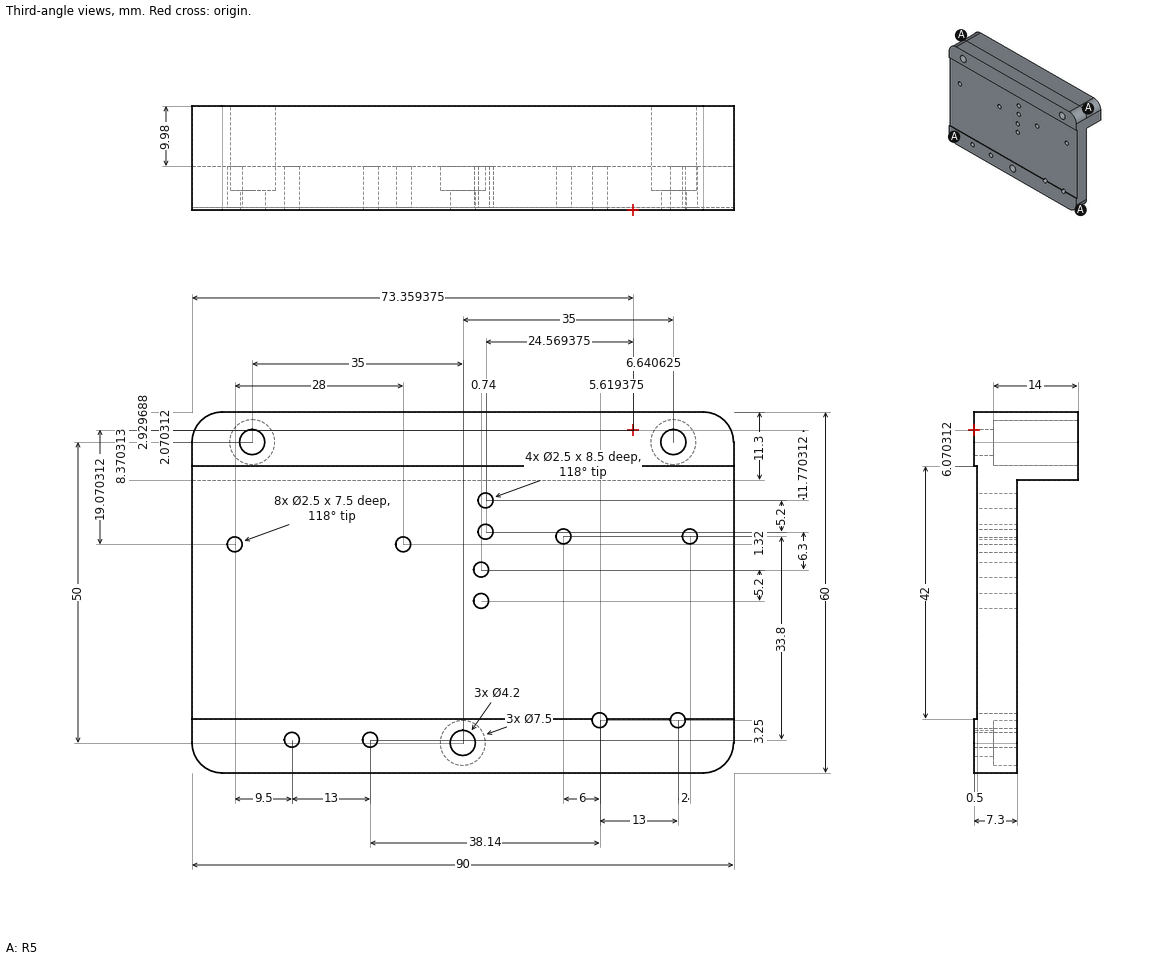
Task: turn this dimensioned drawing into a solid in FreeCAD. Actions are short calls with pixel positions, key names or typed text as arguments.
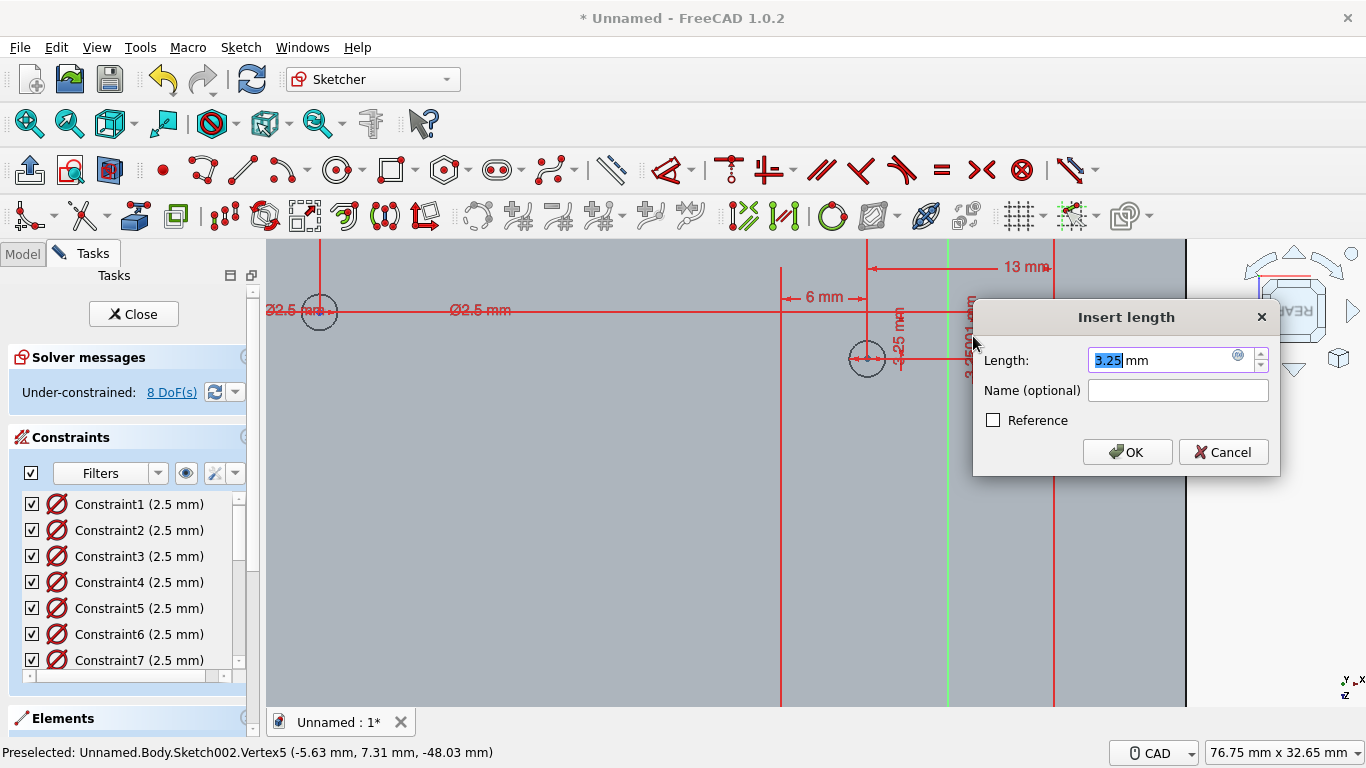
text(3.25)
key(Return)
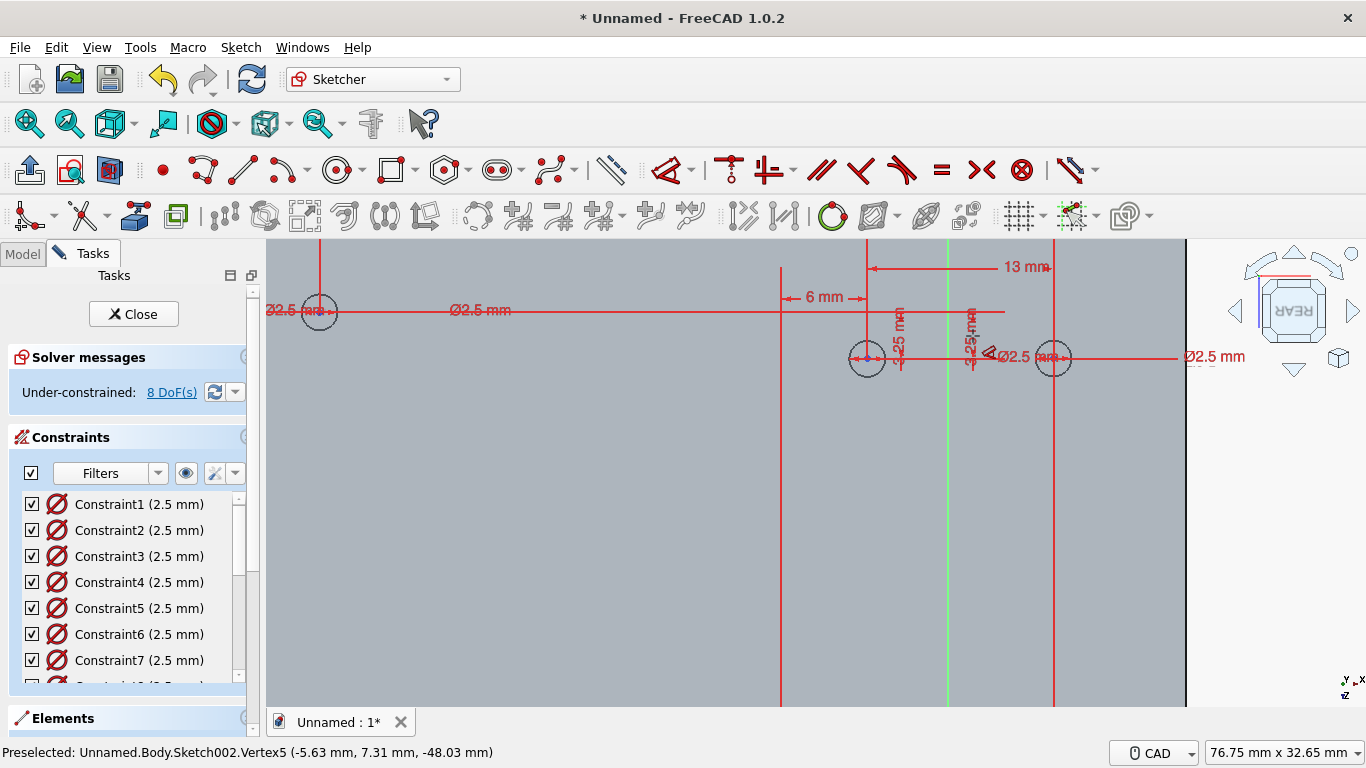
click(320, 312)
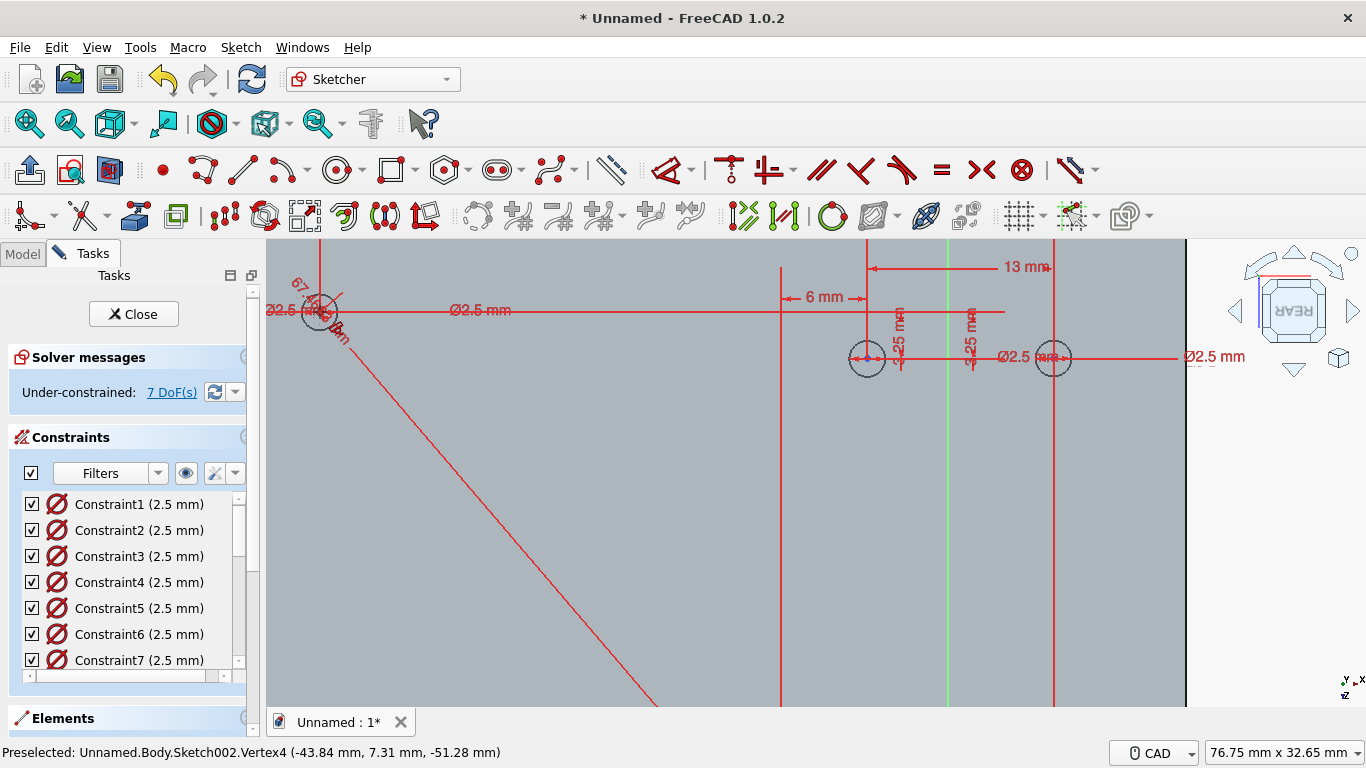
click(1054, 359)
click(1088, 335)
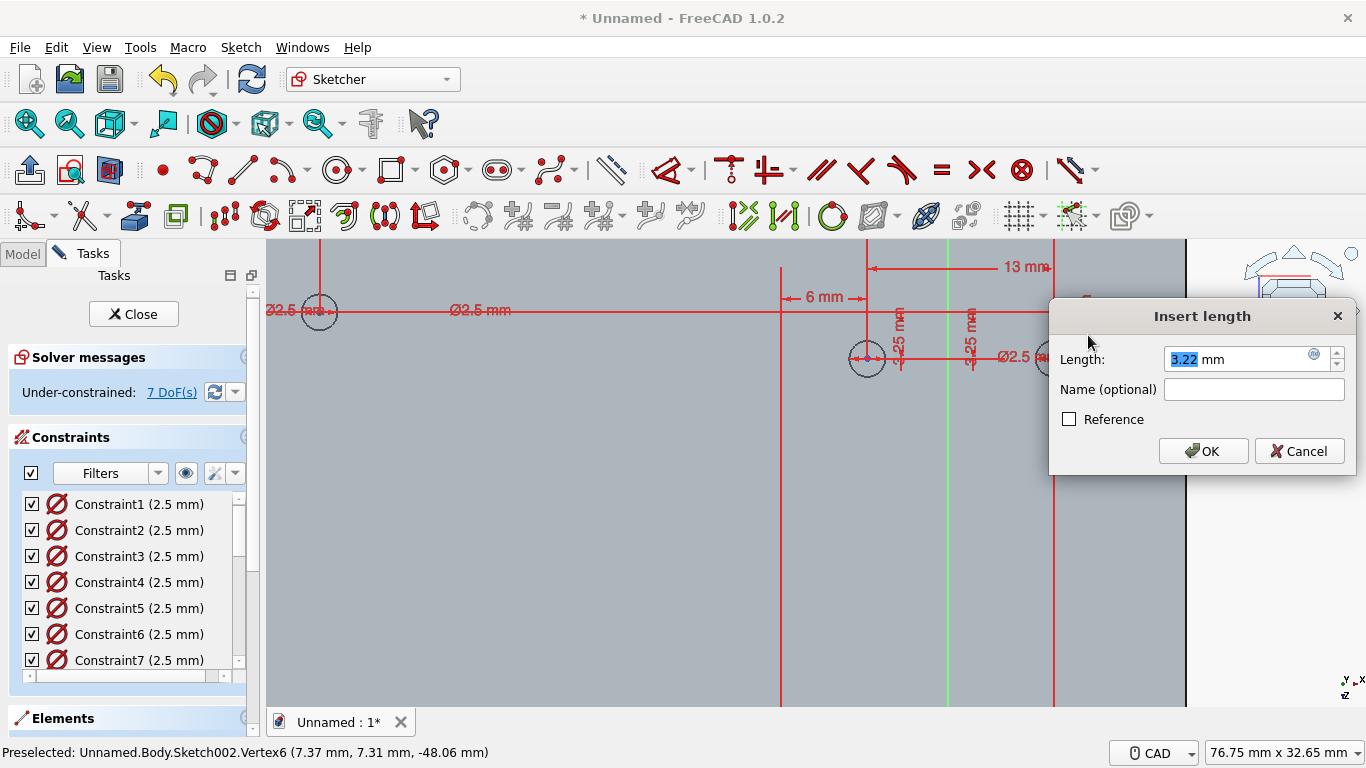
text(3.25)
key(Return)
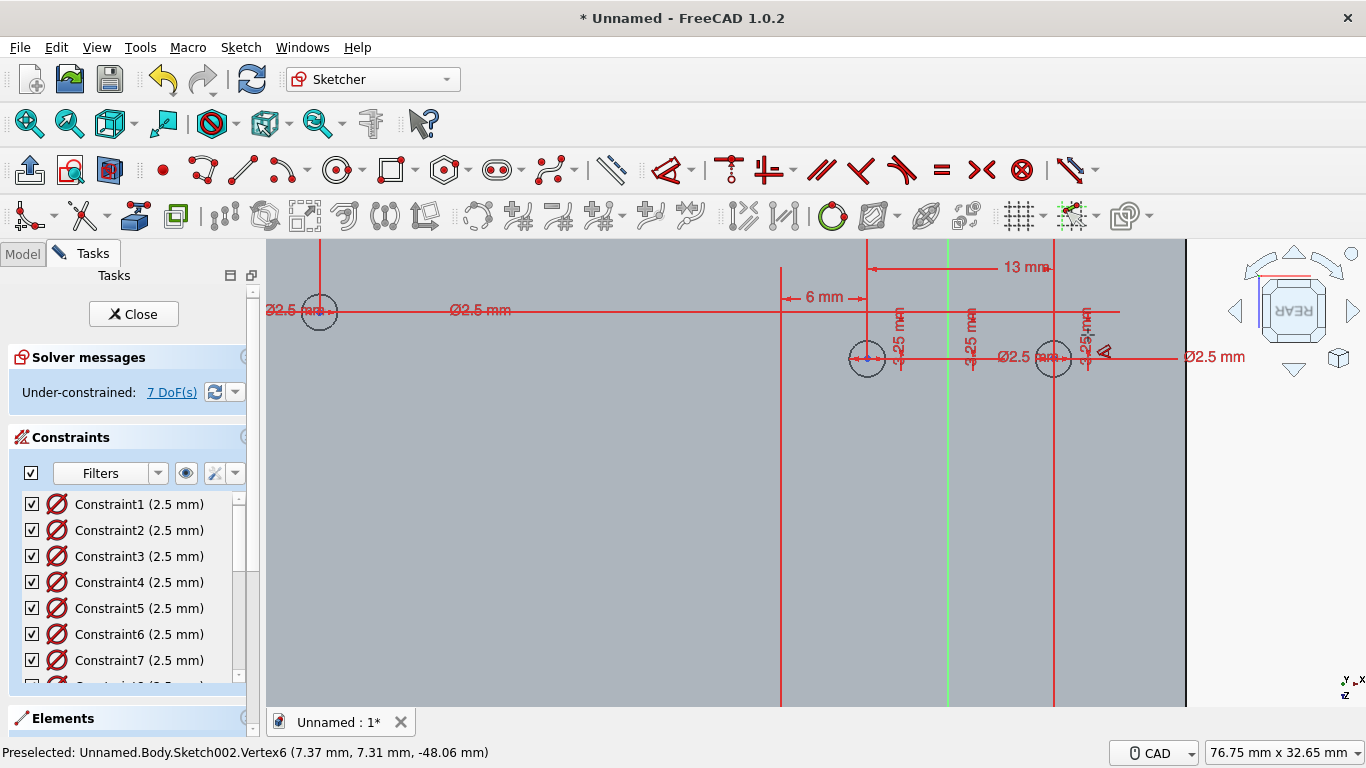
scroll(868, 359, down, 5)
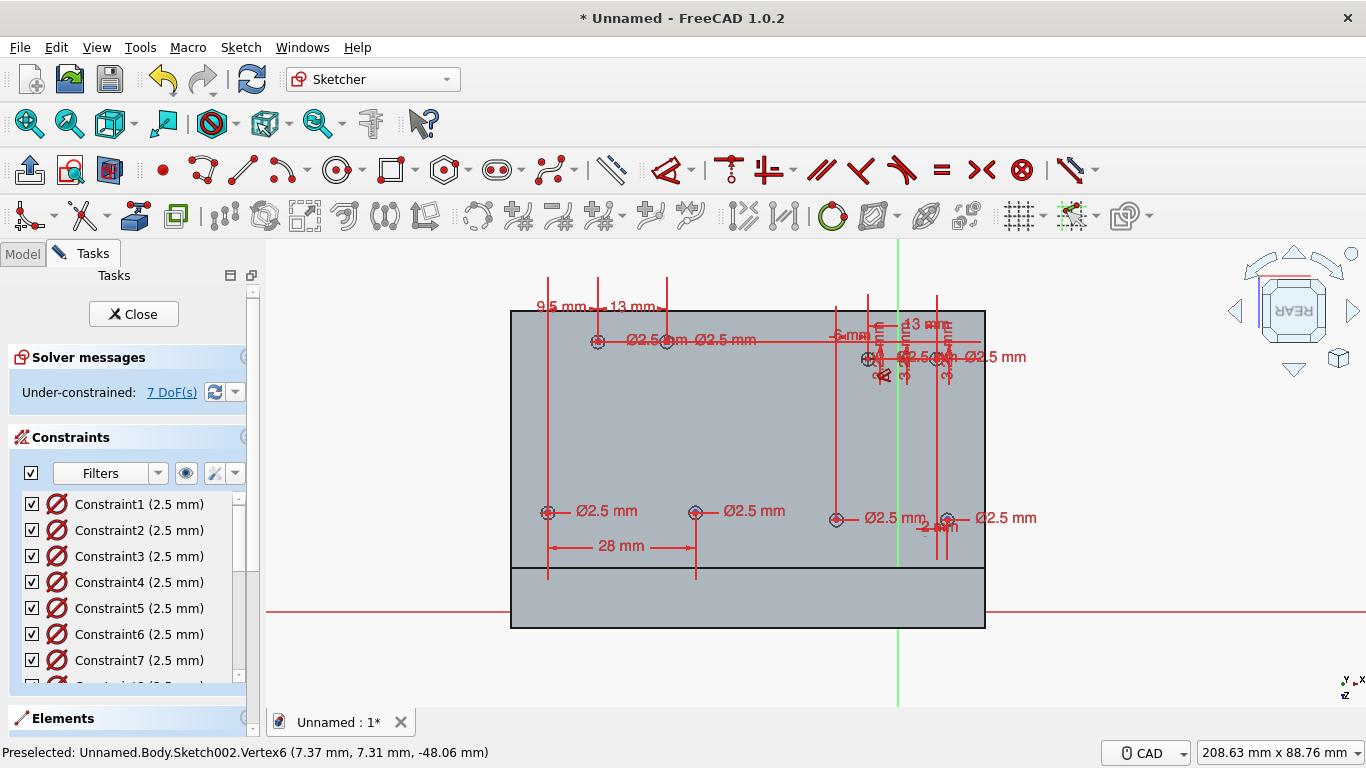
scroll(696, 513, up, 9)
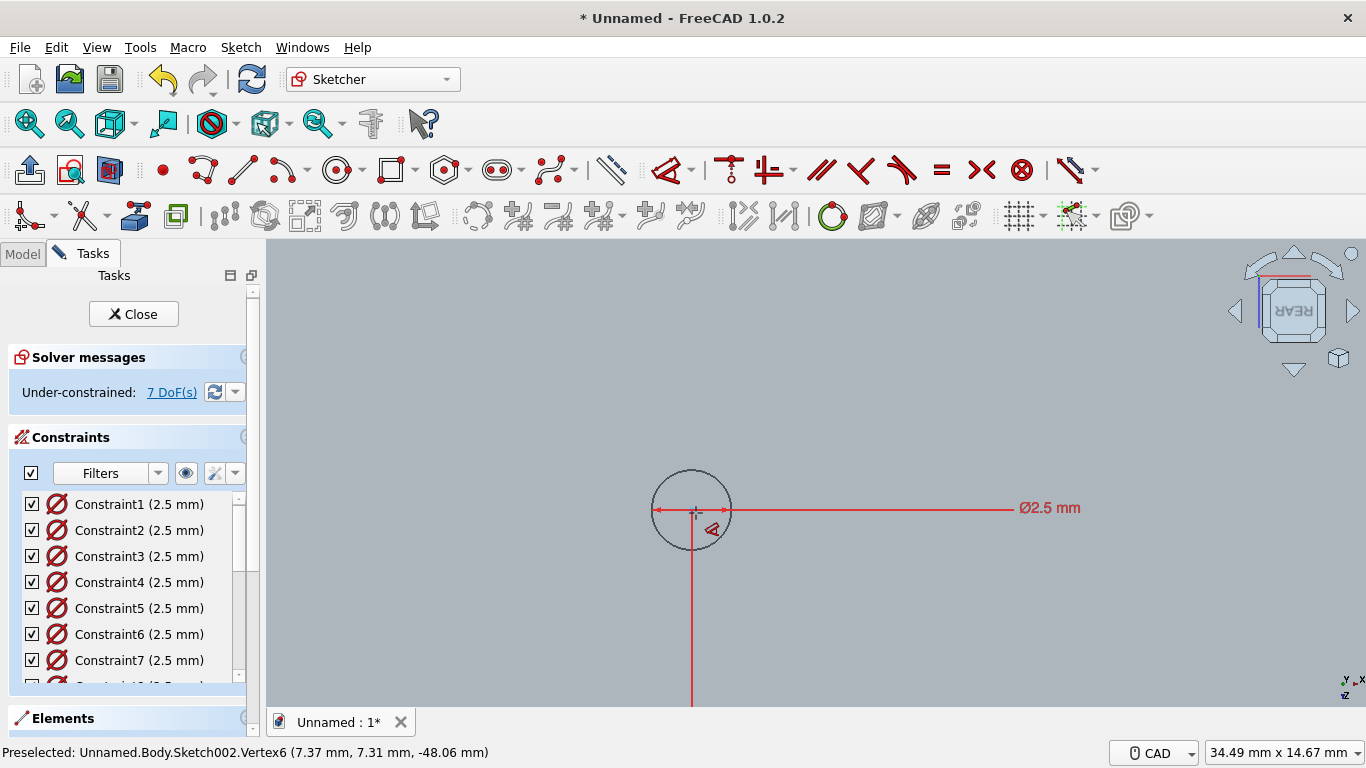
click(692, 510)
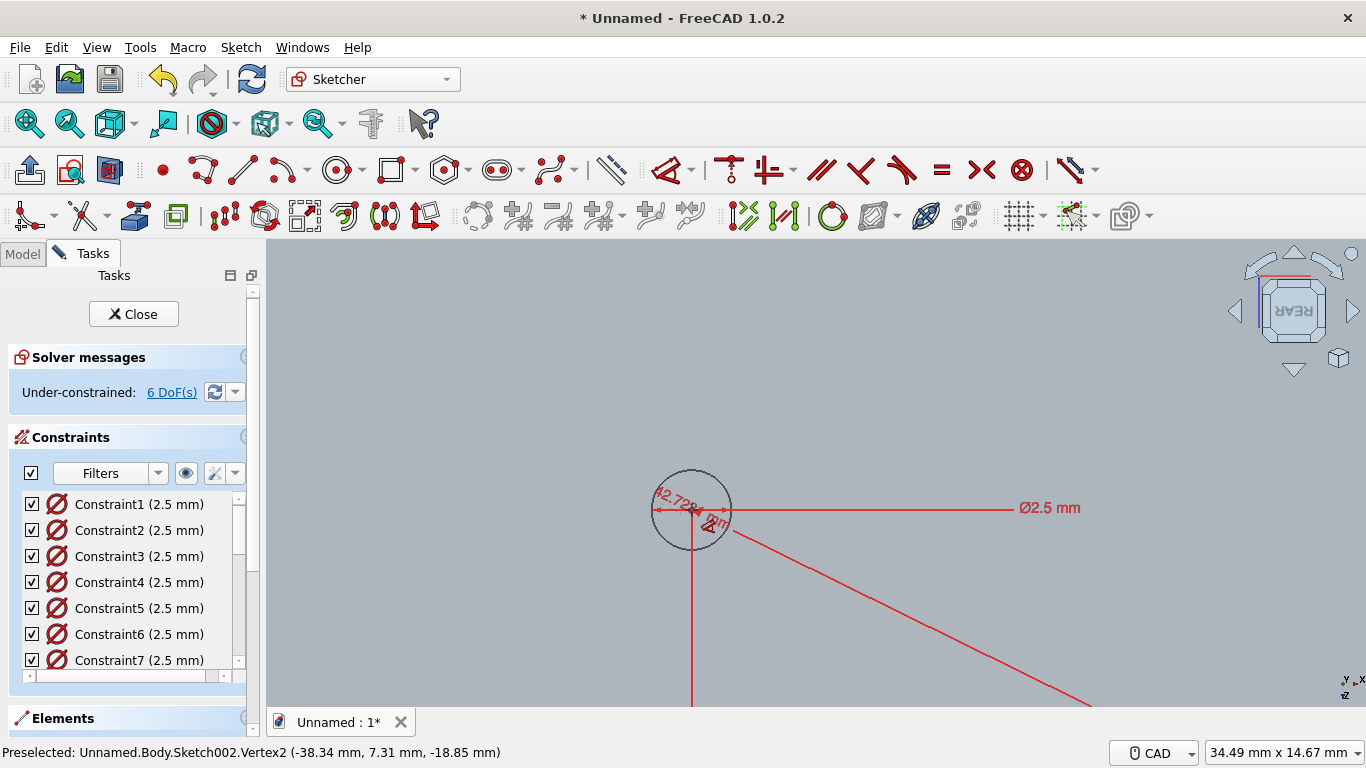
scroll(696, 513, down, 9)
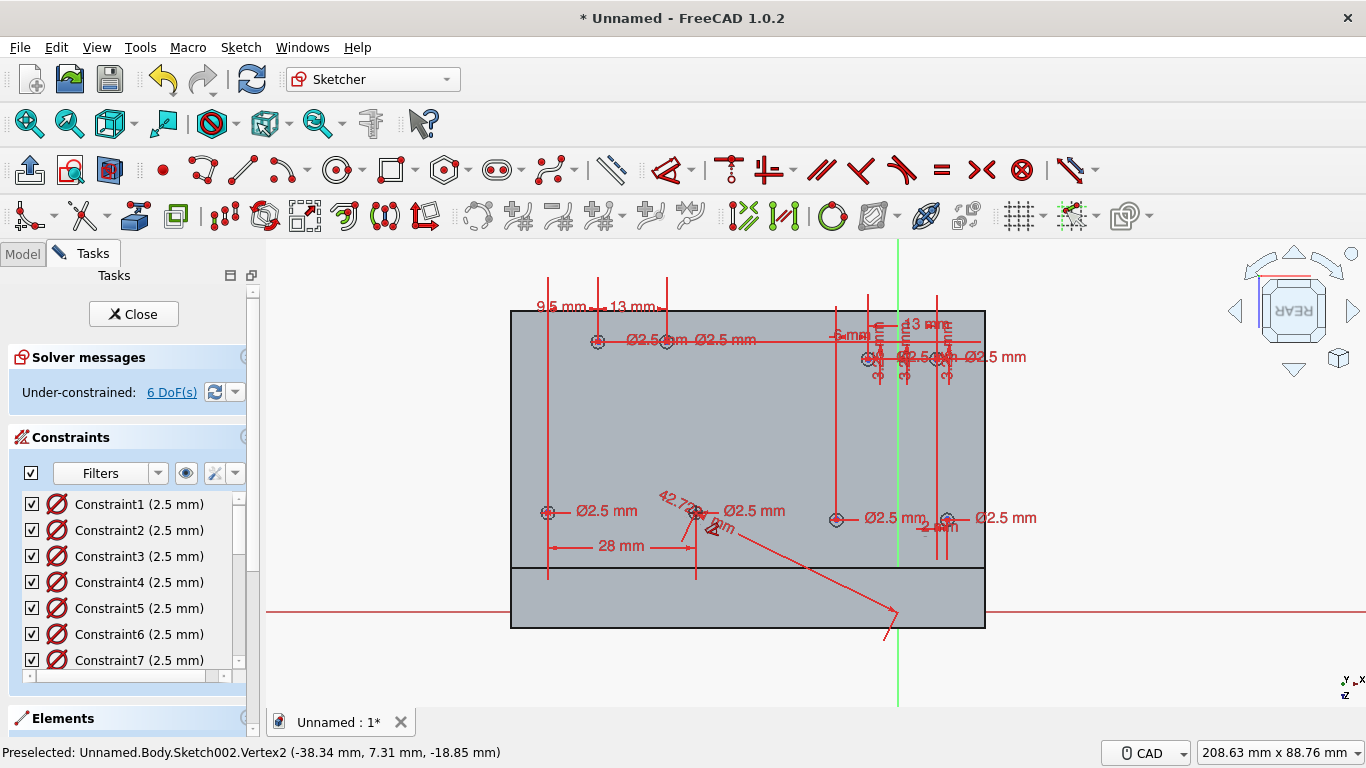
scroll(836, 520, up, 9)